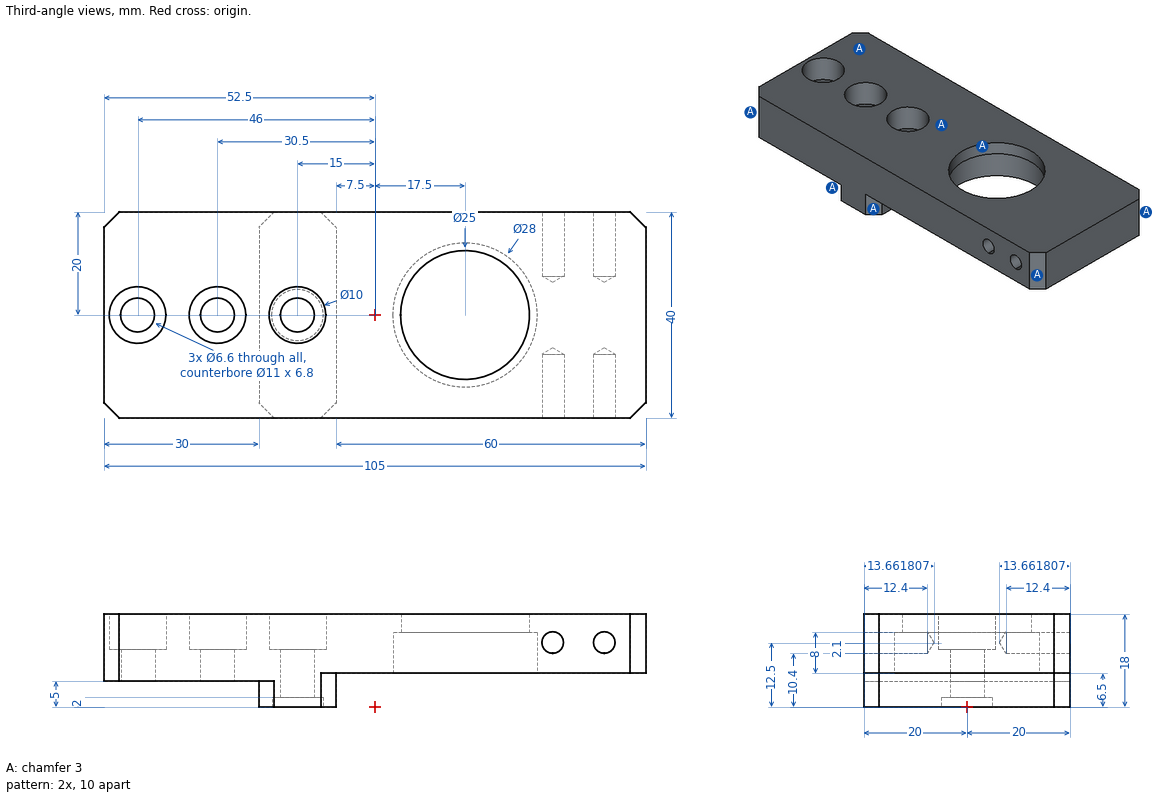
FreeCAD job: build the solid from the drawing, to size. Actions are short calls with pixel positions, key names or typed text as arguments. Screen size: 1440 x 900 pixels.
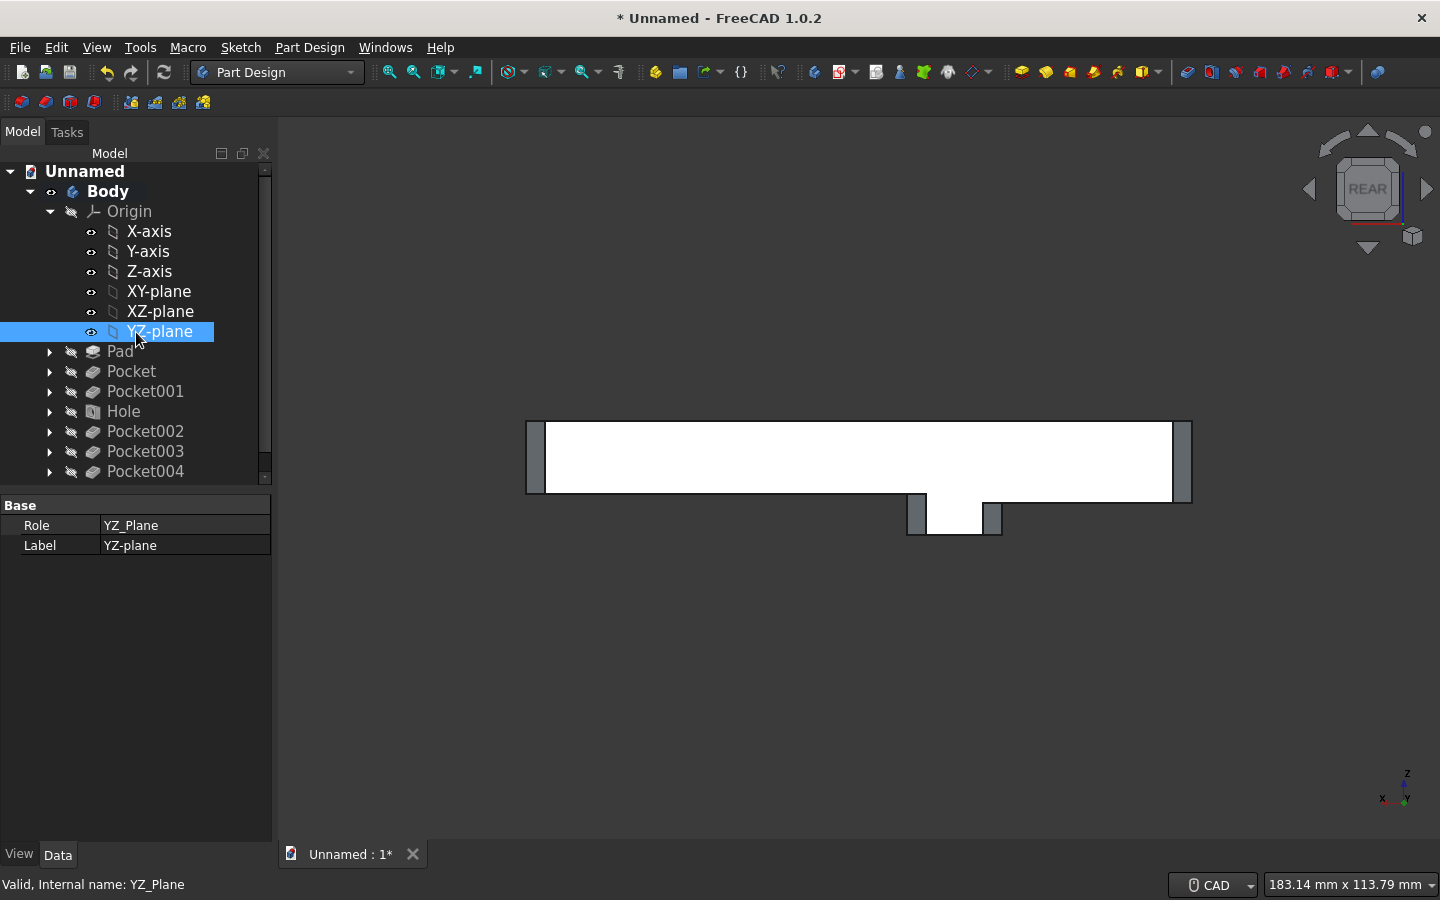
click(972, 72)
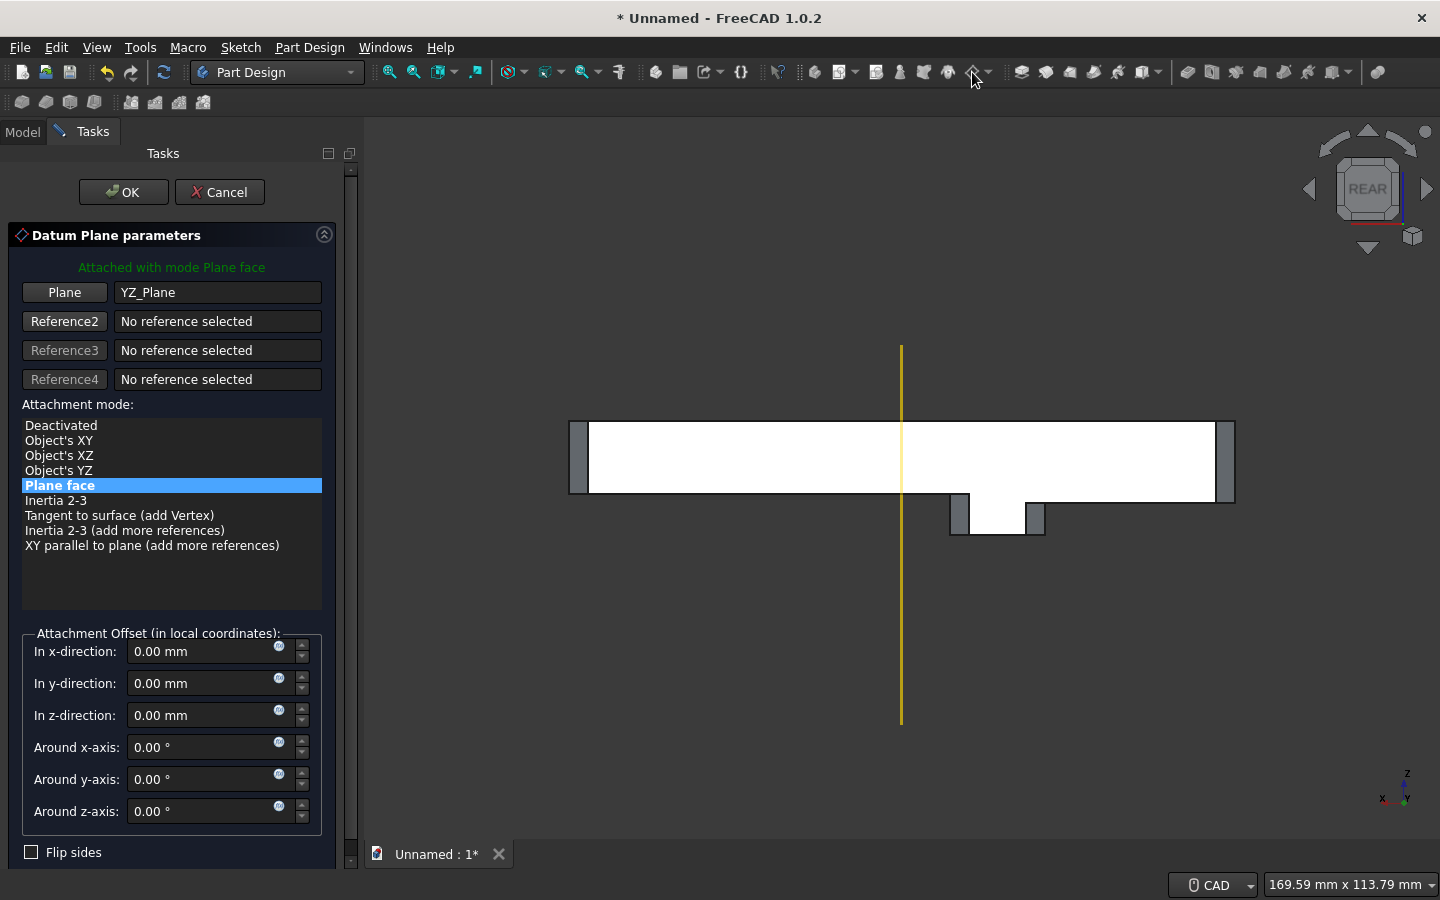
triple_click(210, 715)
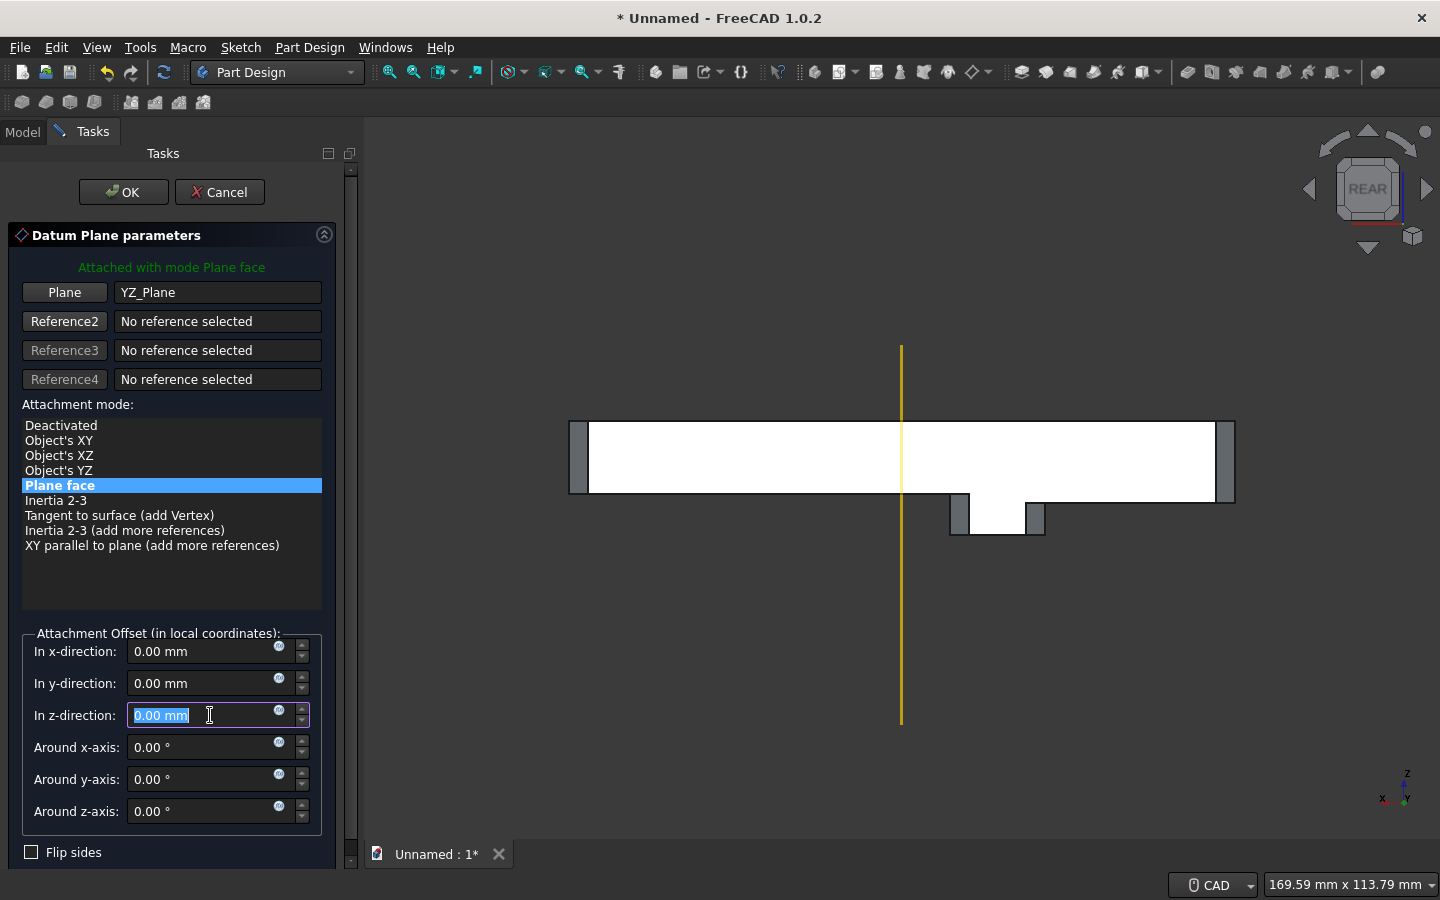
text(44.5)
key(Tab)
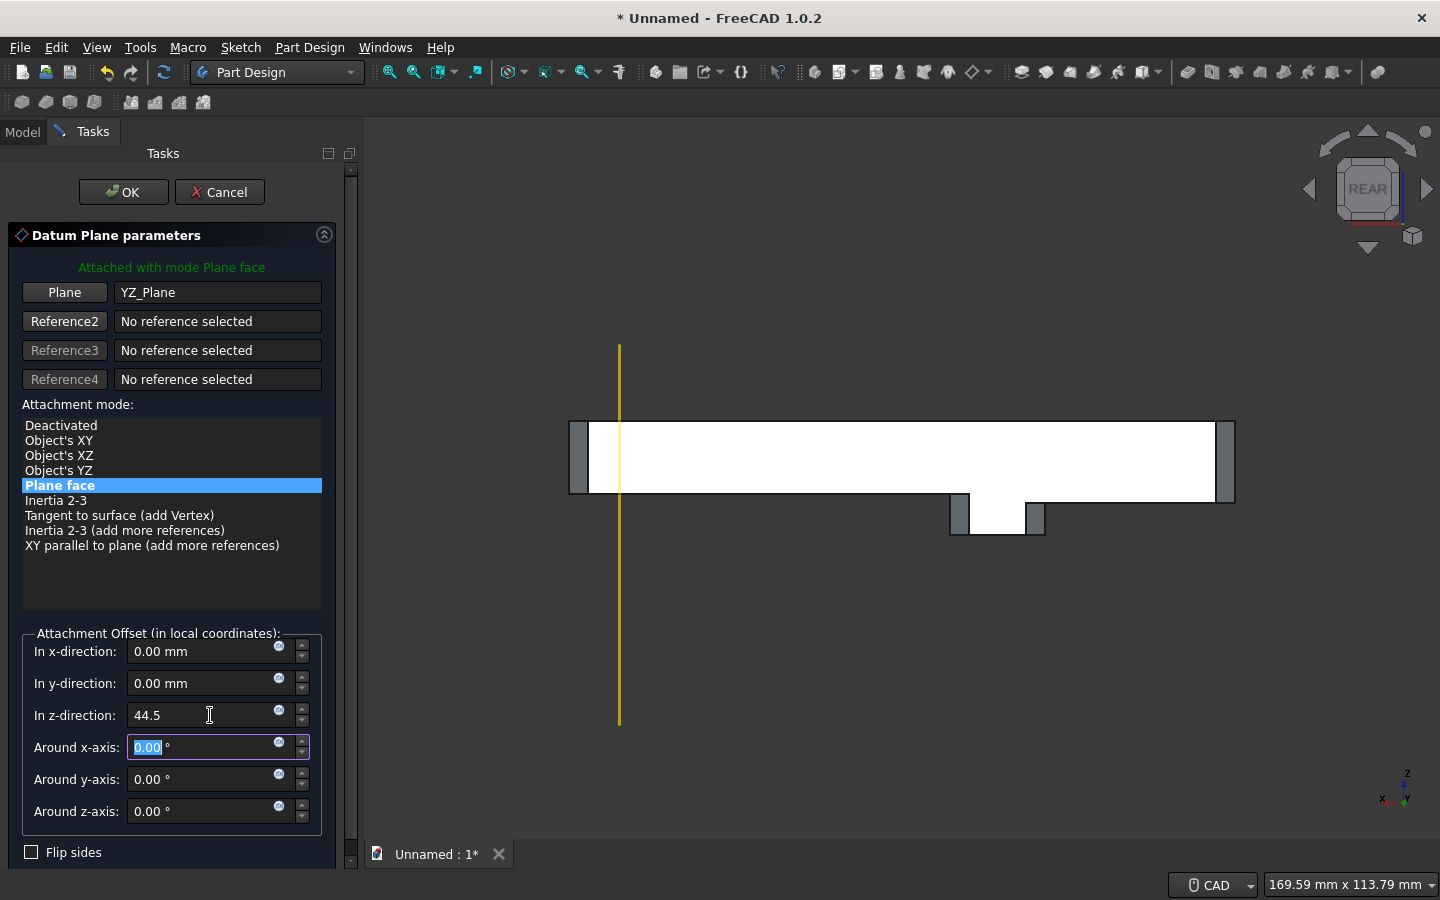
click(124, 192)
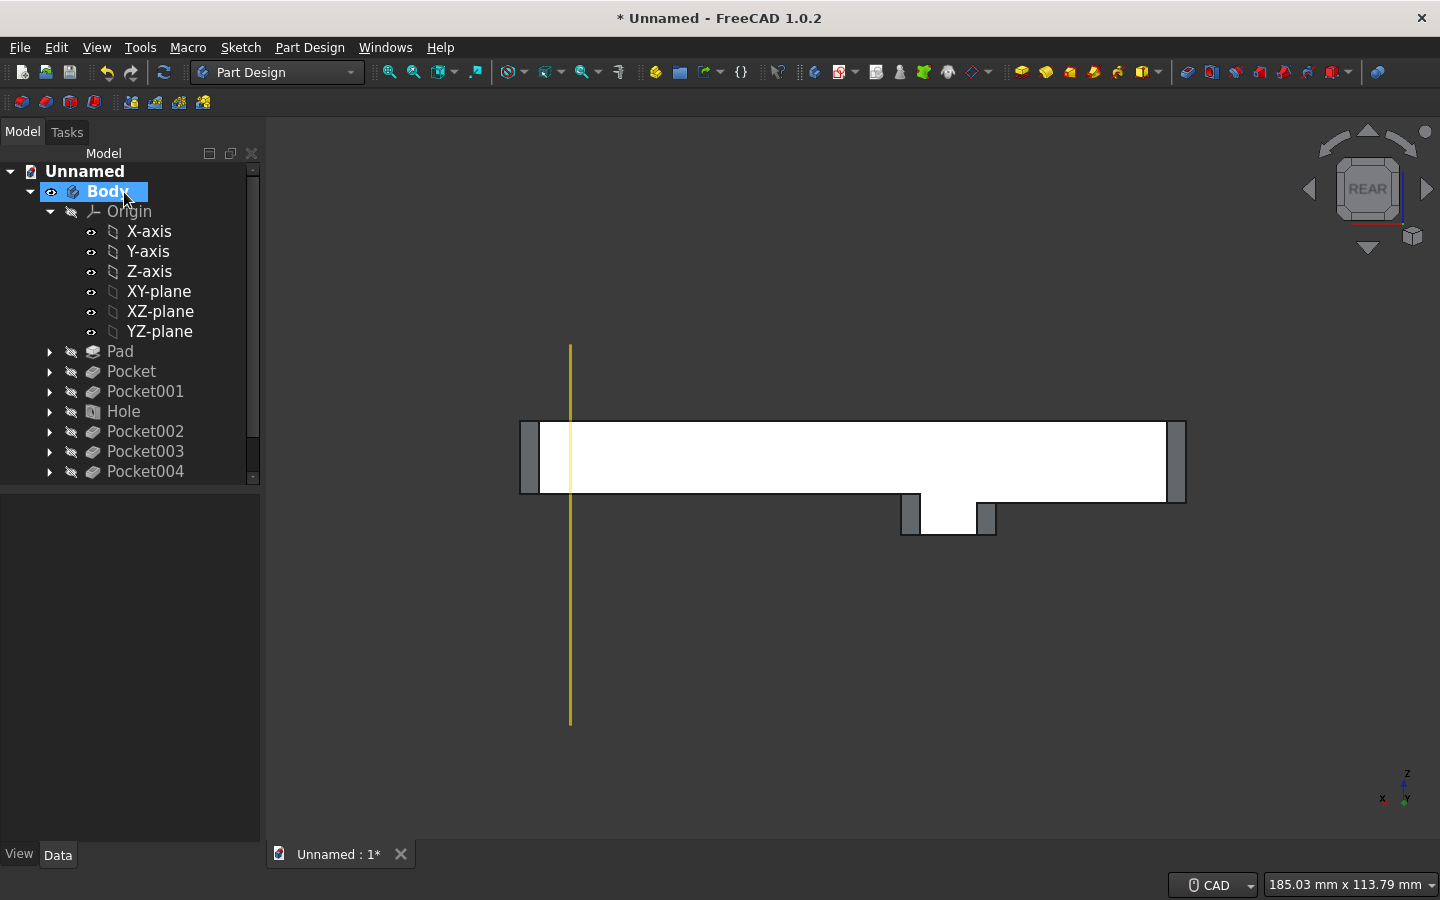
scroll(100, 327, down, 3)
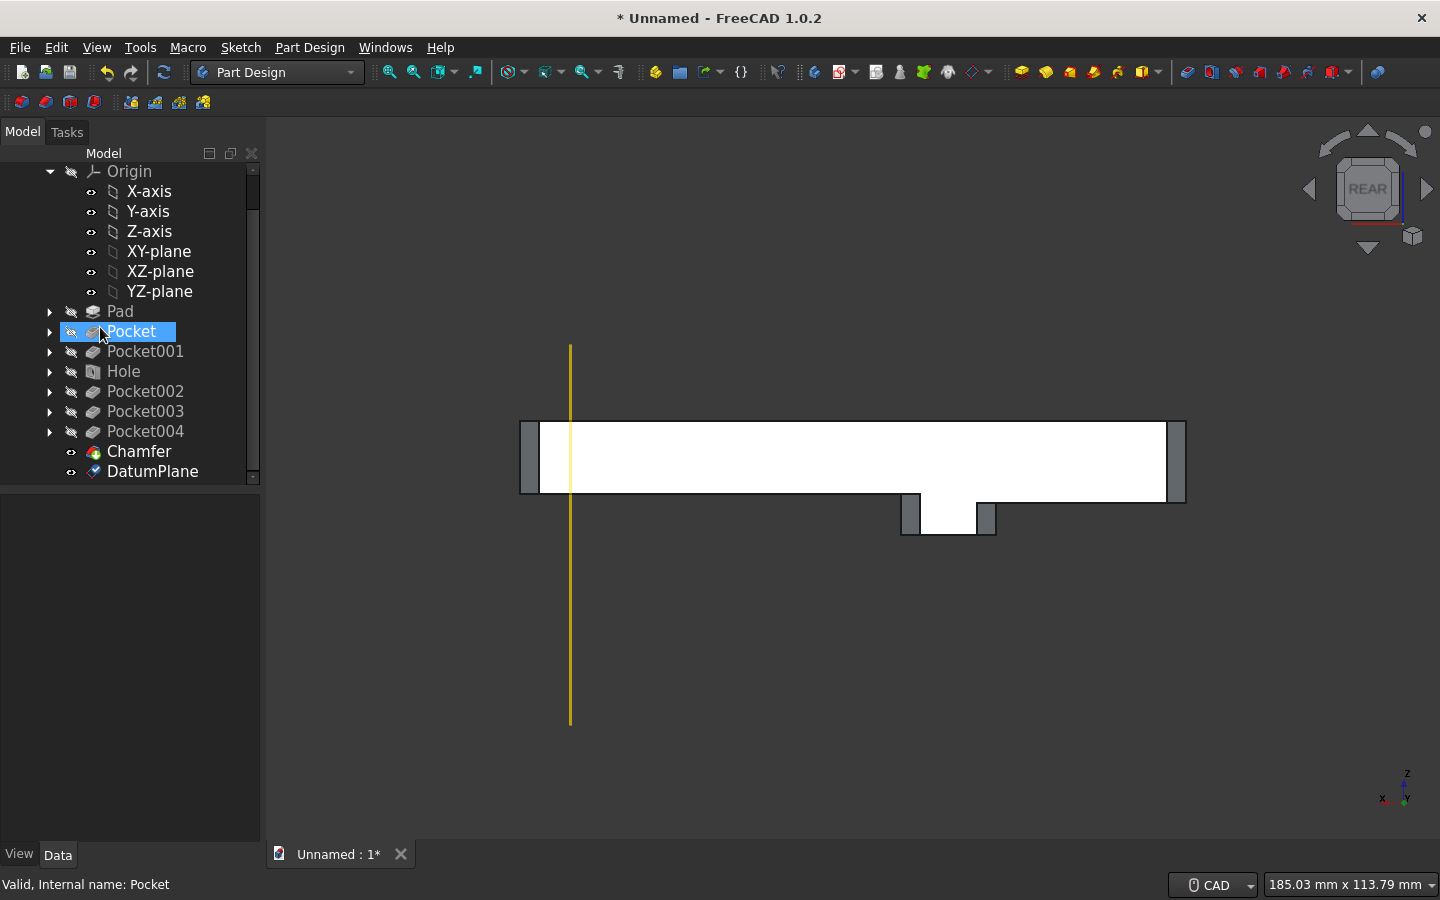
click(116, 472)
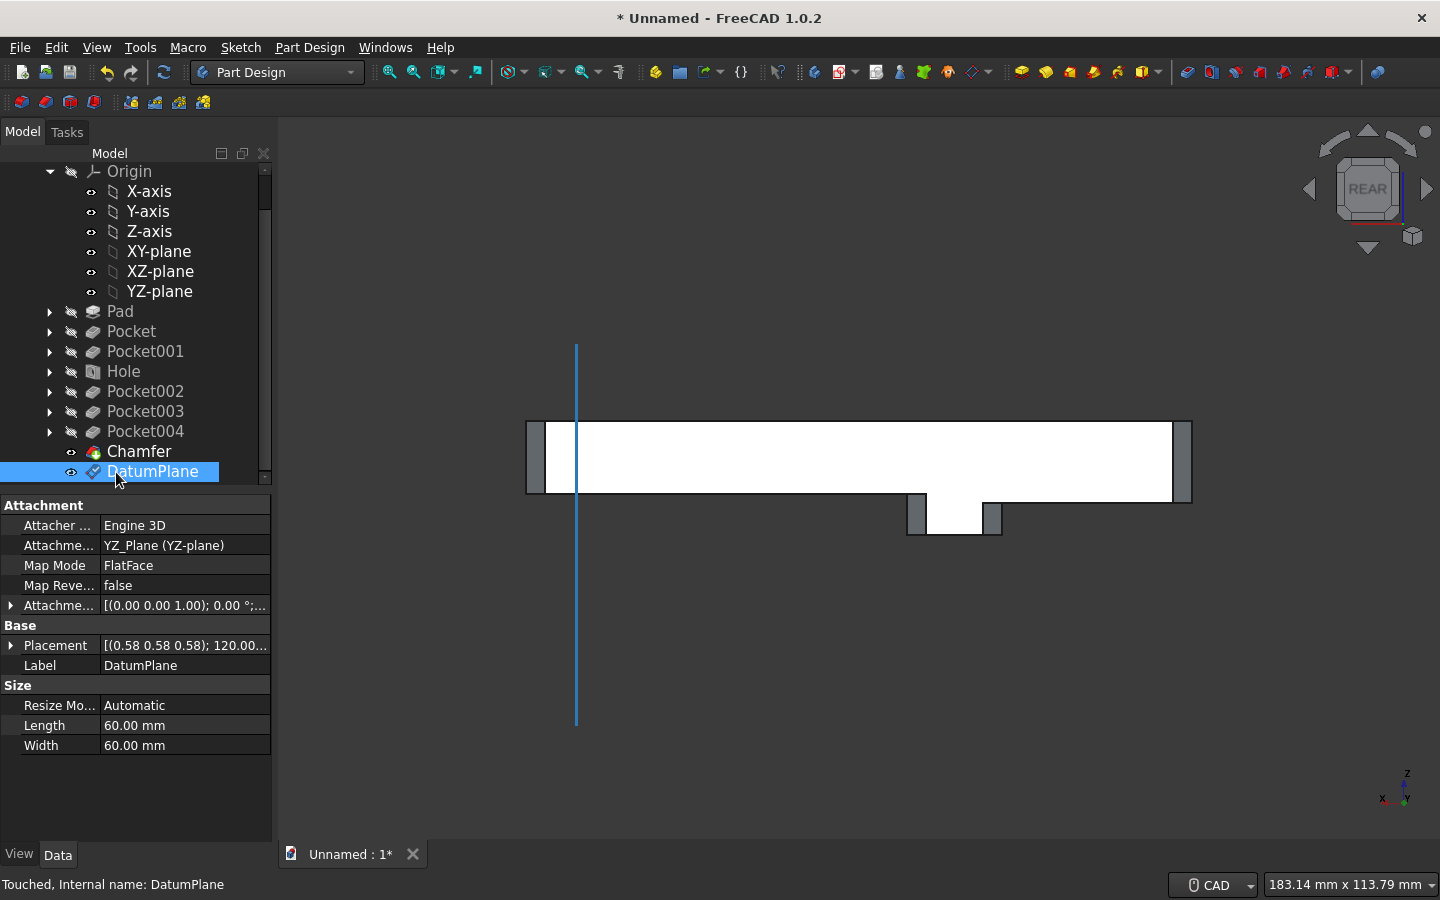
click(840, 72)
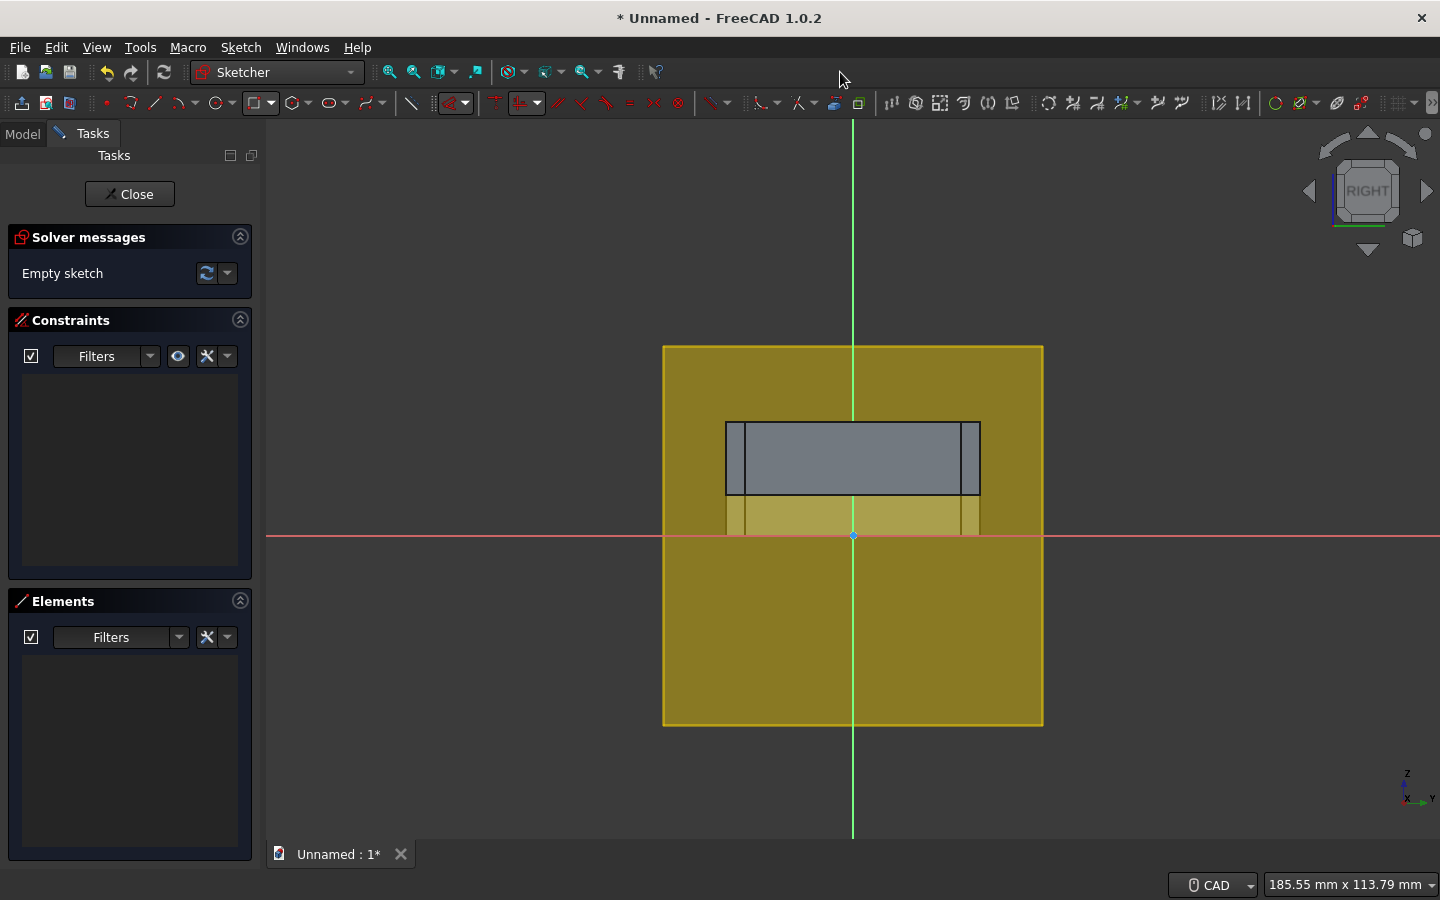
click(70, 104)